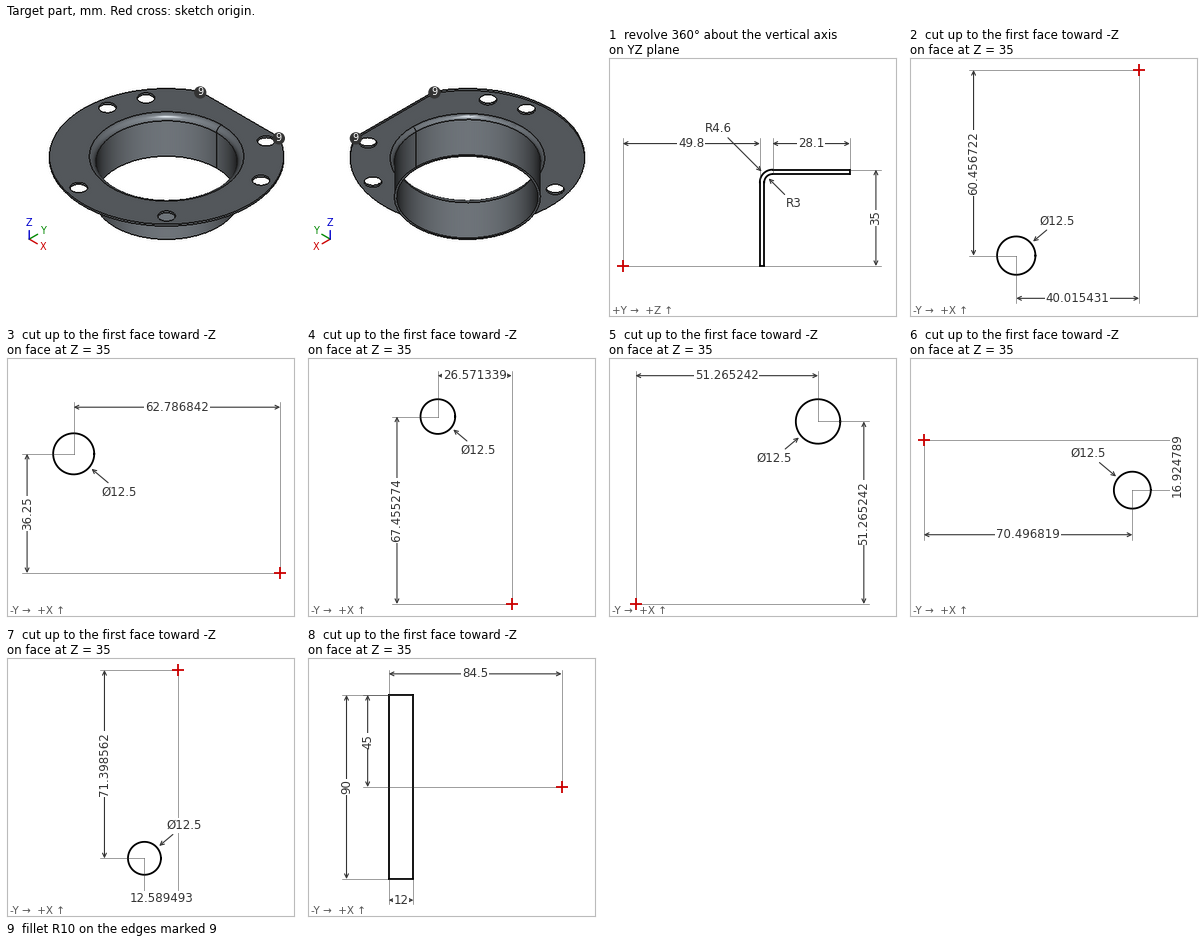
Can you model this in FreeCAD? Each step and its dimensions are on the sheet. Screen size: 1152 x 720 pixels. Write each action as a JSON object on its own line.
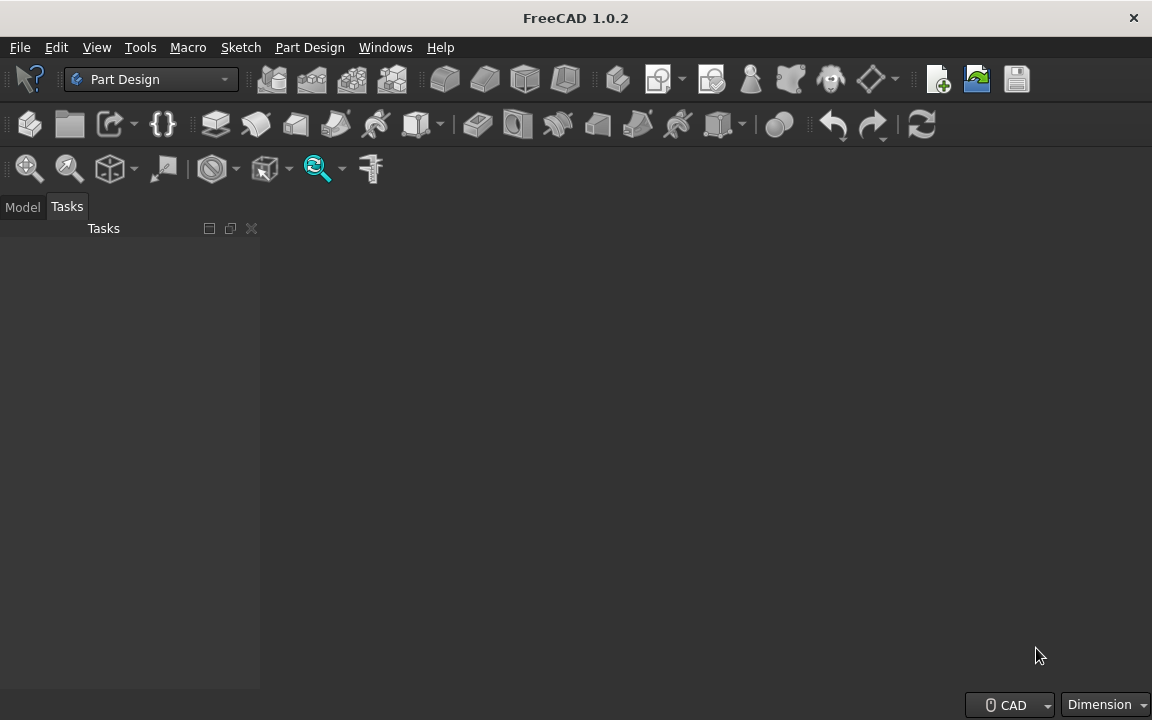
{"action": "key", "text": "ctrl+n"}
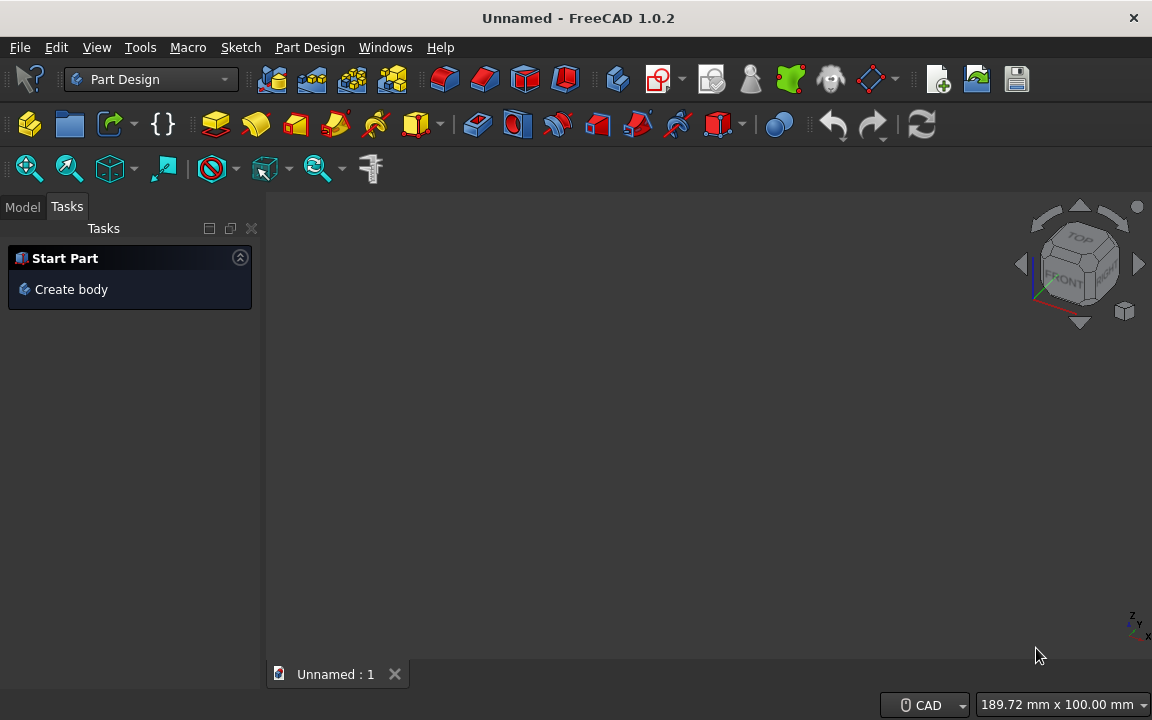
{"action": "left_click", "coordinate": [658, 80]}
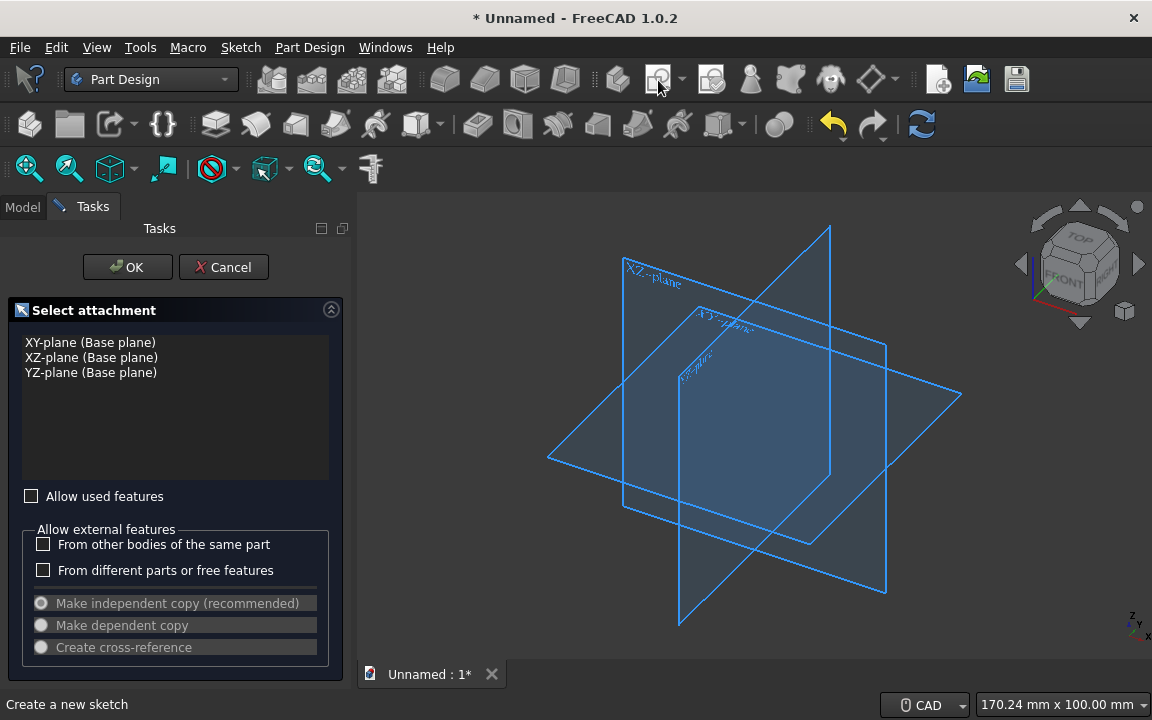
{"action": "left_click", "coordinate": [82, 372]}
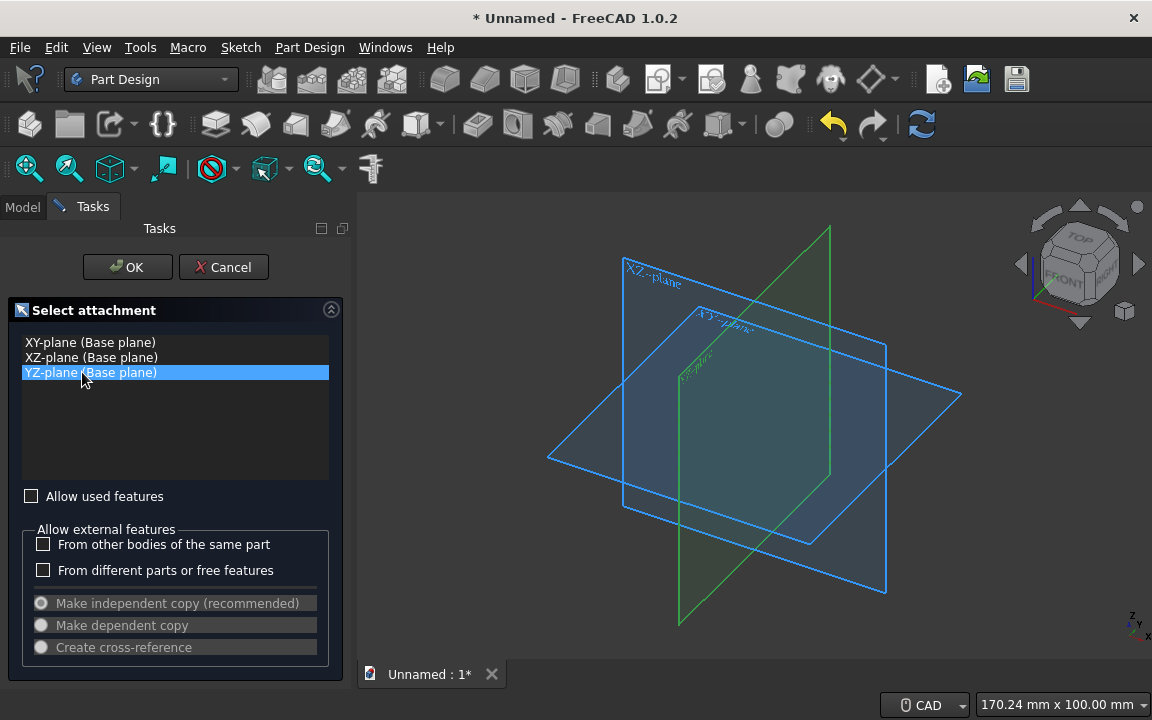
{"action": "left_click", "coordinate": [128, 267]}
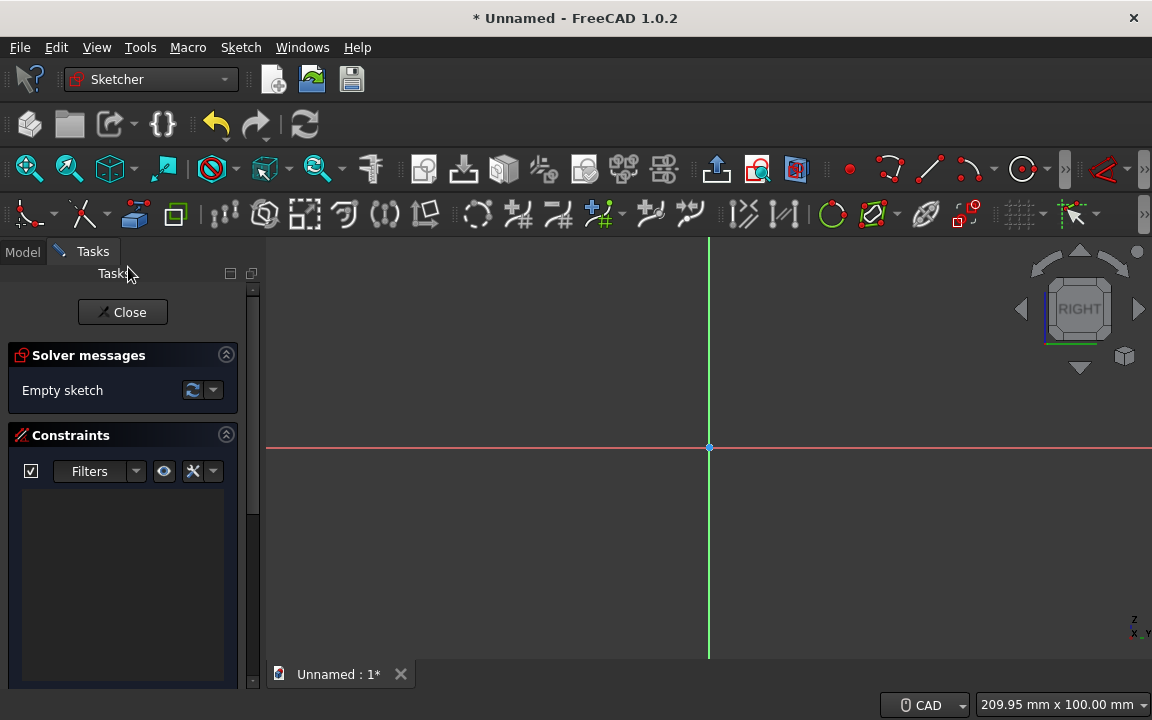
{"action": "scroll", "coordinate": [294, 631], "scroll_direction": "down", "scroll_amount": 1}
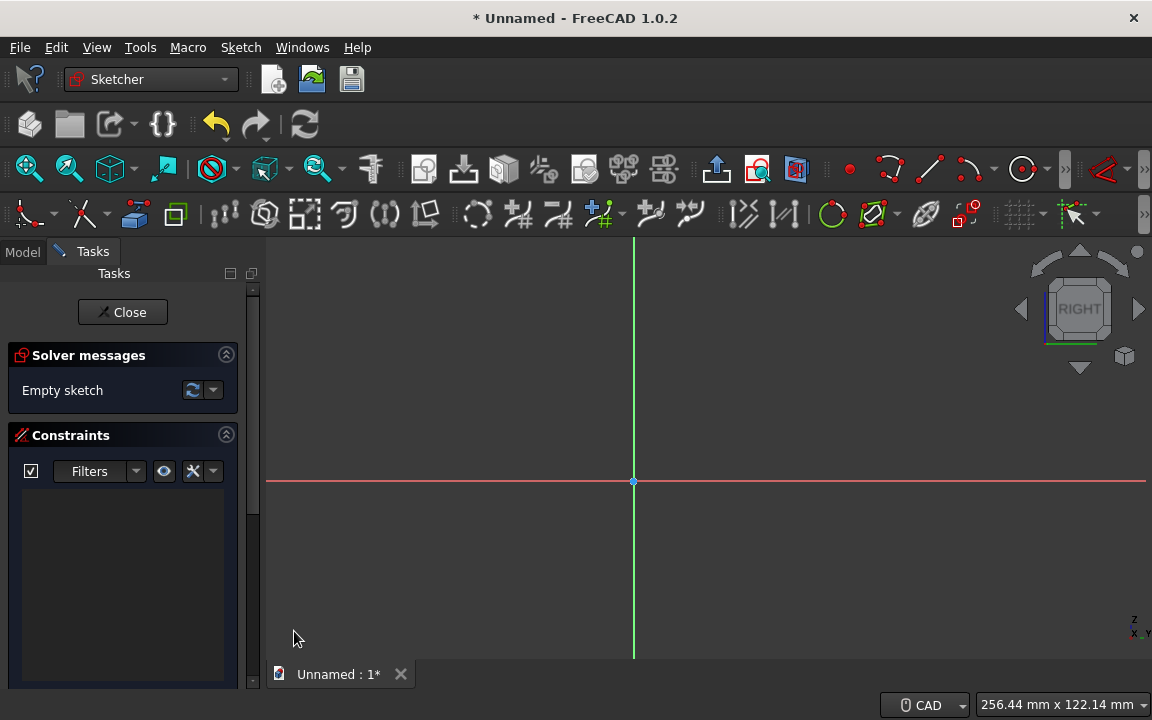
{"action": "scroll", "coordinate": [941, 388], "scroll_direction": "up", "scroll_amount": 3}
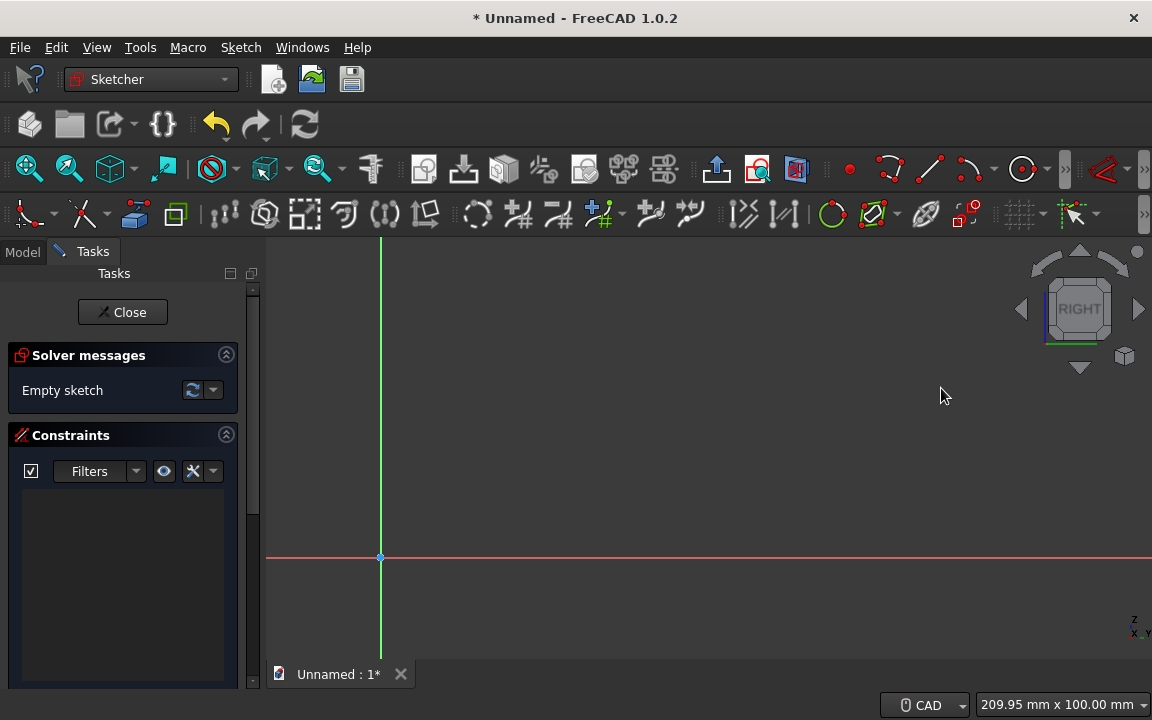
{"action": "key", "text": "g m"}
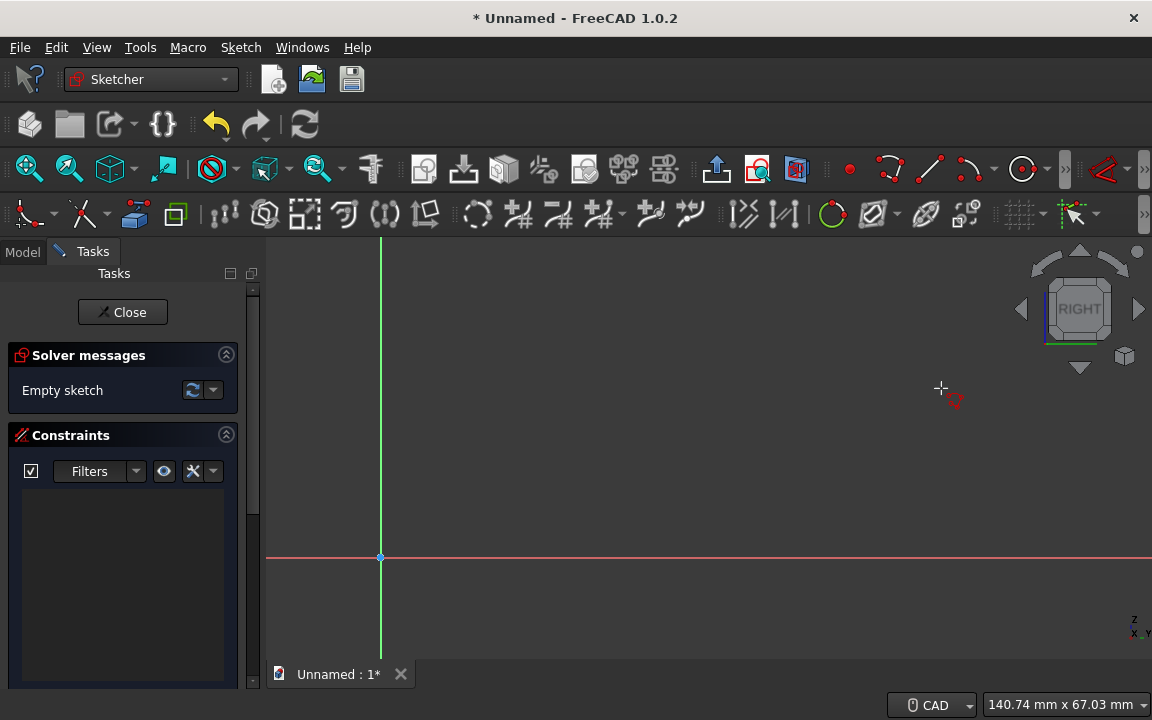
{"action": "left_click", "coordinate": [694, 366]}
{"action": "left_click", "coordinate": [694, 558]}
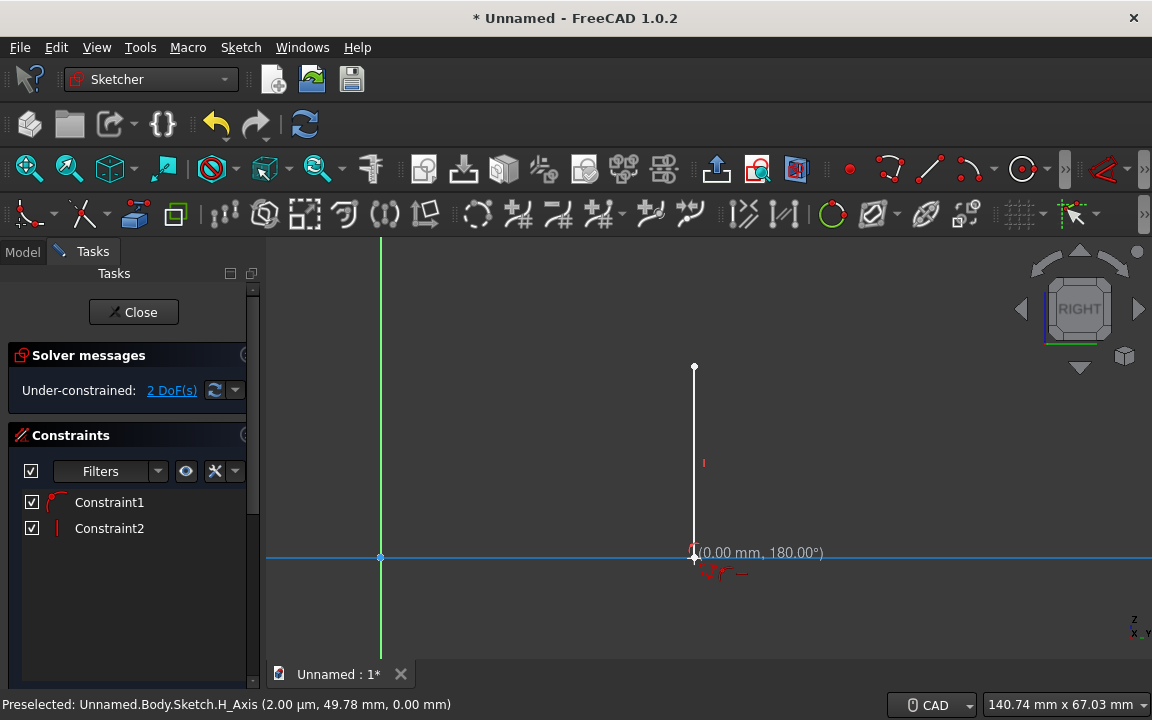
{"action": "scroll", "coordinate": [704, 558], "scroll_direction": "up", "scroll_amount": 3}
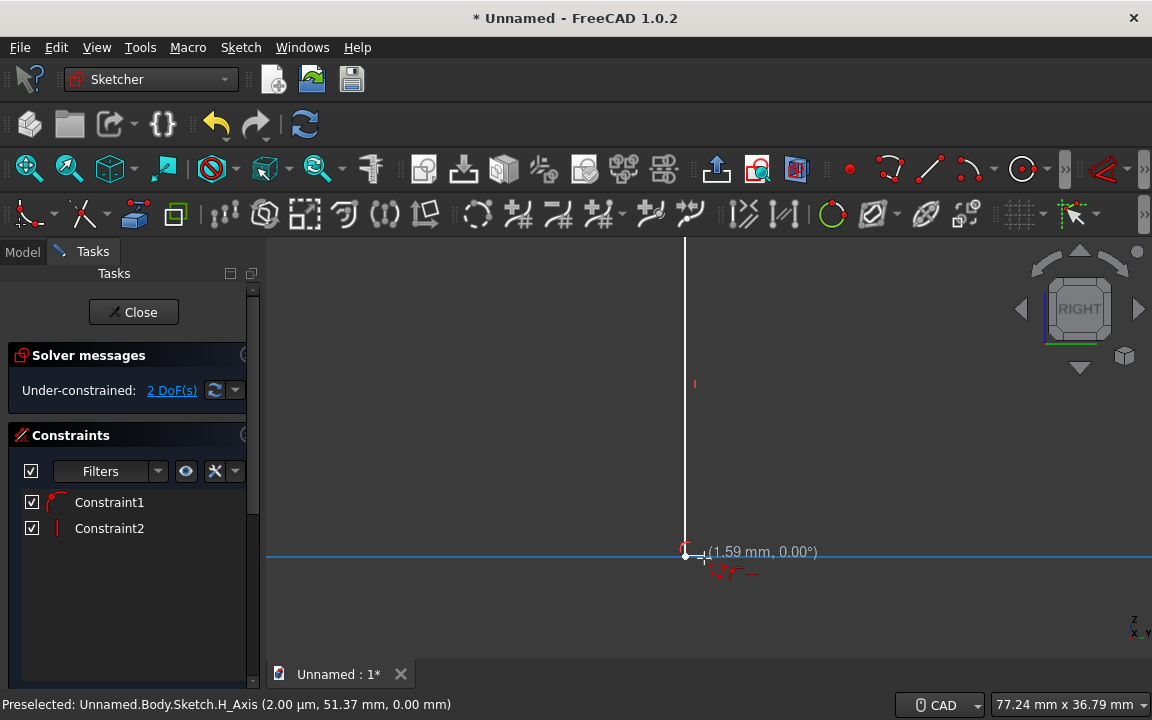
{"action": "left_click", "coordinate": [704, 548]}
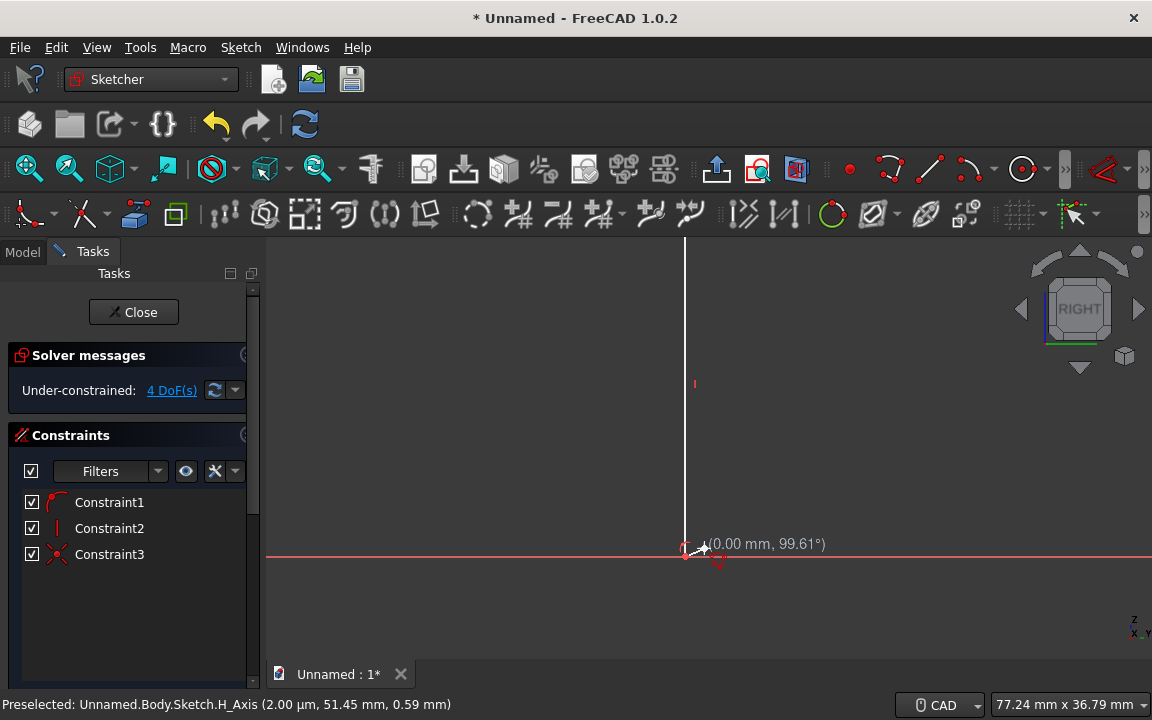
{"action": "scroll", "coordinate": [705, 560], "scroll_direction": "down", "scroll_amount": 3}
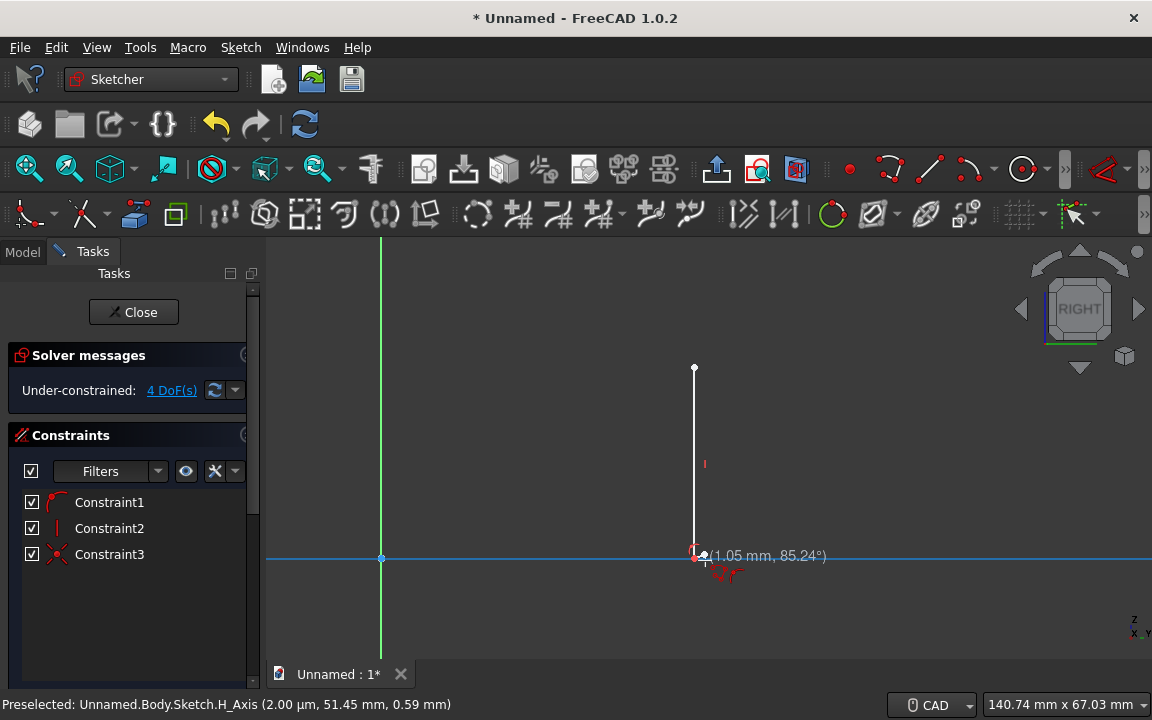
{"action": "scroll", "coordinate": [705, 367], "scroll_direction": "up", "scroll_amount": 3}